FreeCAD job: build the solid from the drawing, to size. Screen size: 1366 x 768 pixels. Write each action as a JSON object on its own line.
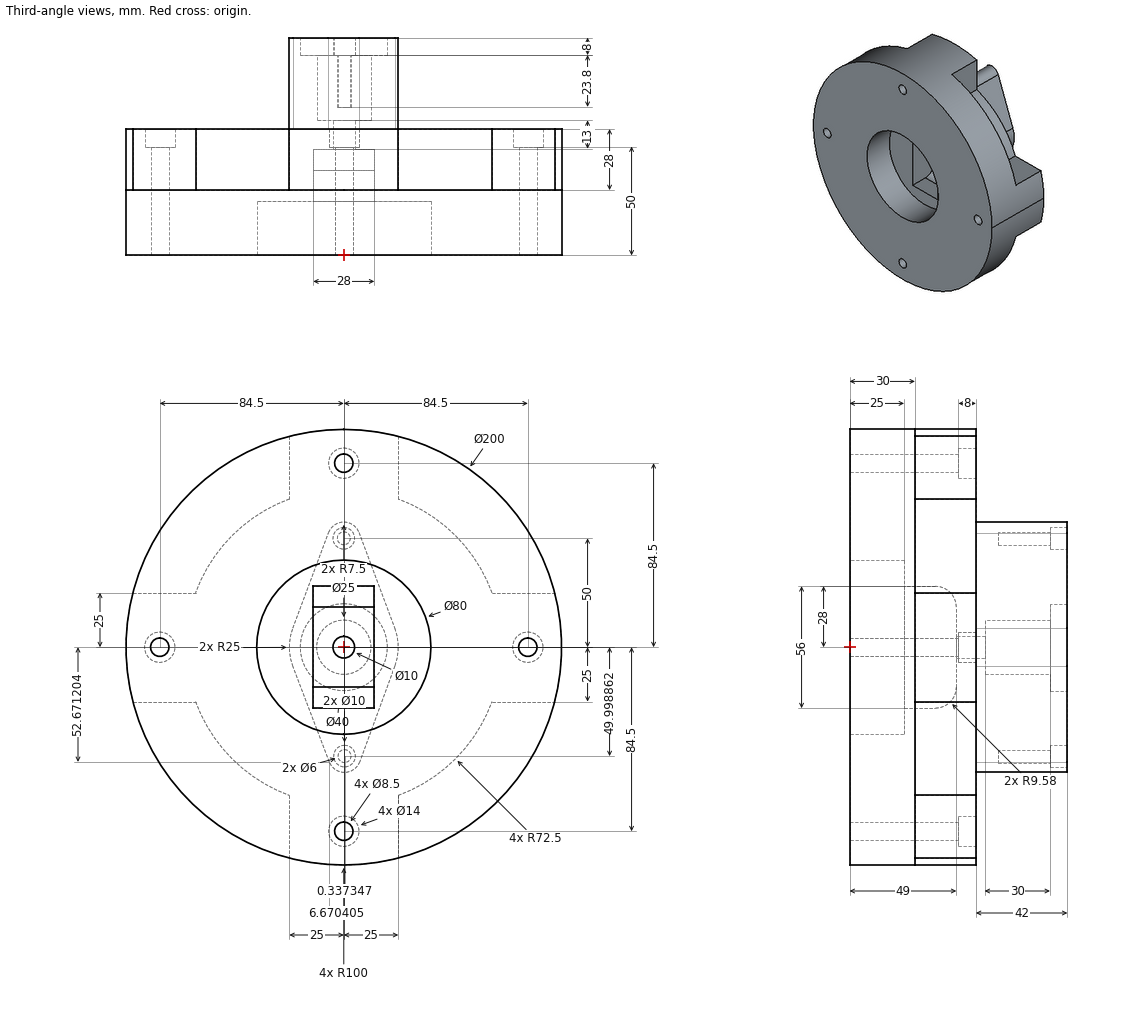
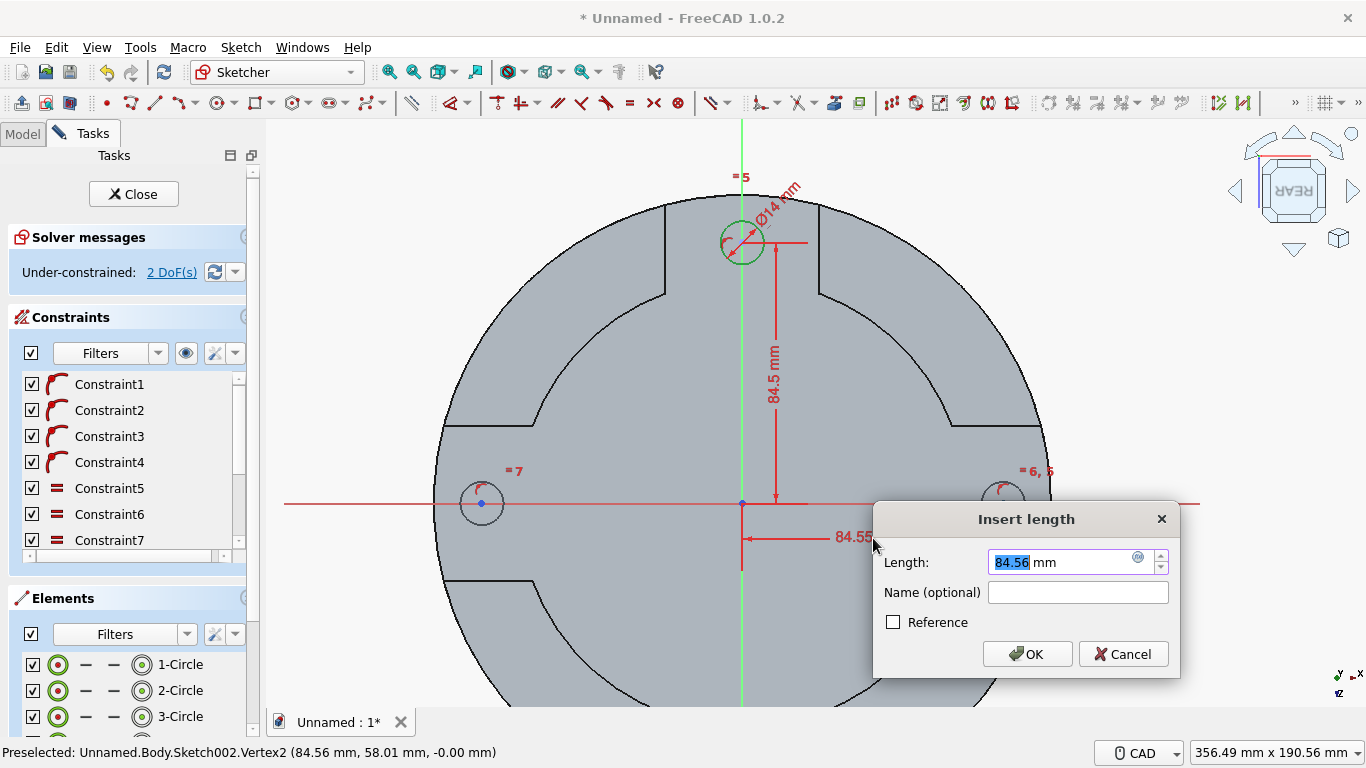
{"action": "type", "text": "84.5"}
{"action": "key", "text": "Return"}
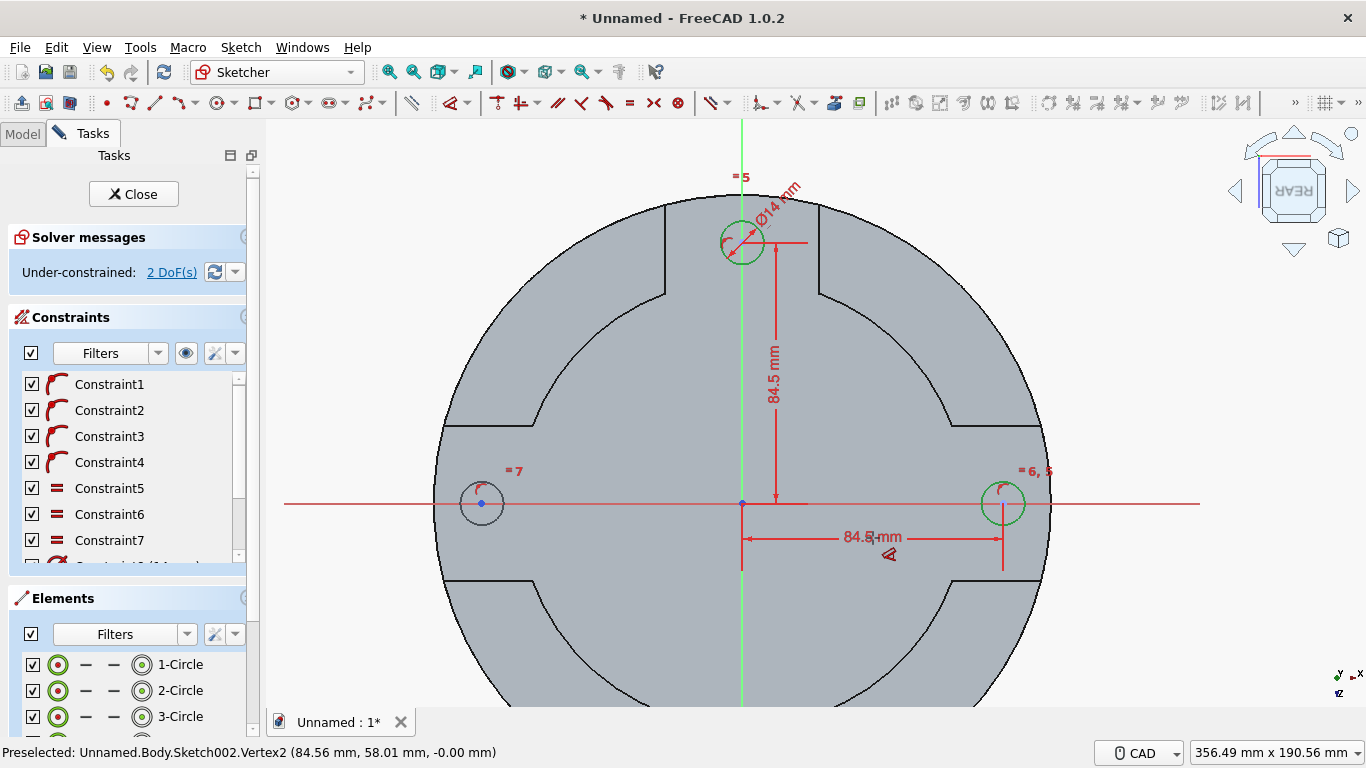
{"action": "scroll", "coordinate": [758, 229], "scroll_direction": "down", "scroll_amount": 2}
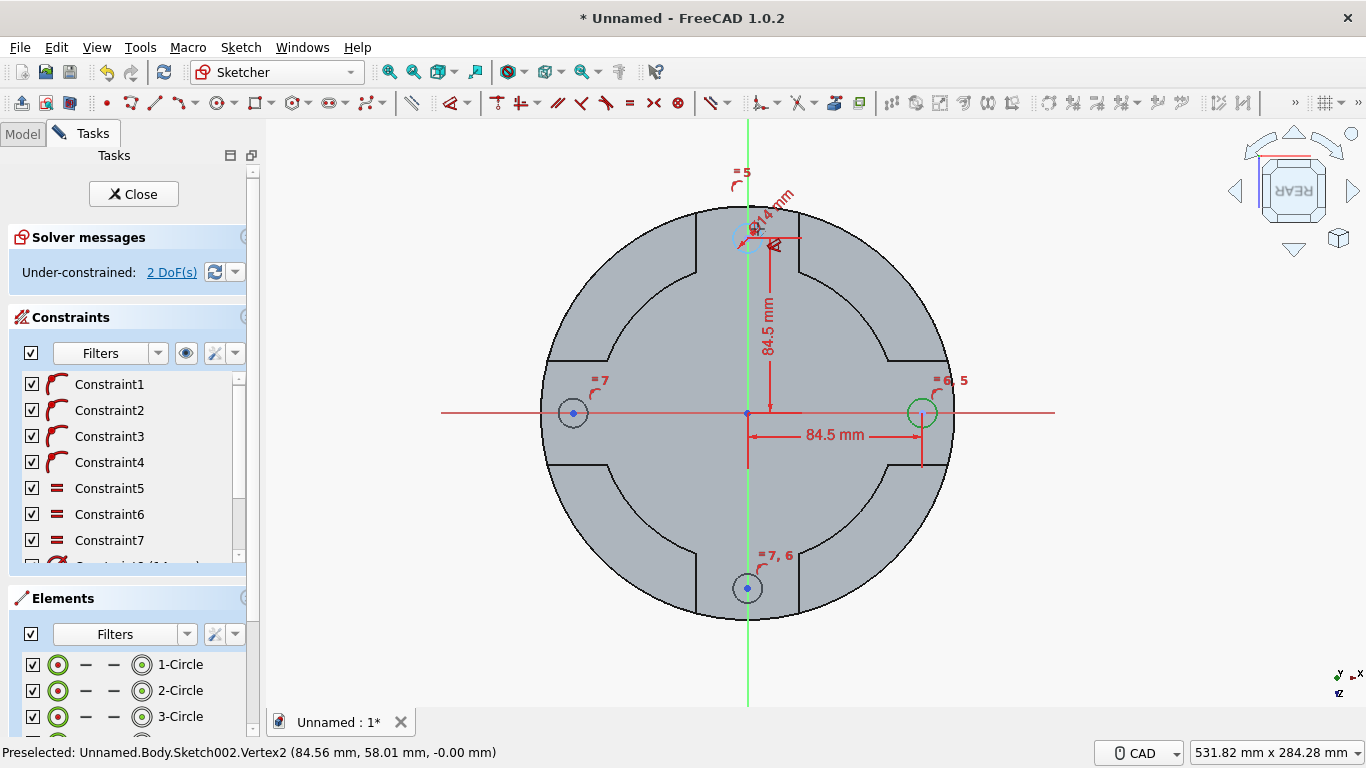
{"action": "left_click", "coordinate": [748, 588]}
{"action": "left_click", "coordinate": [782, 501]}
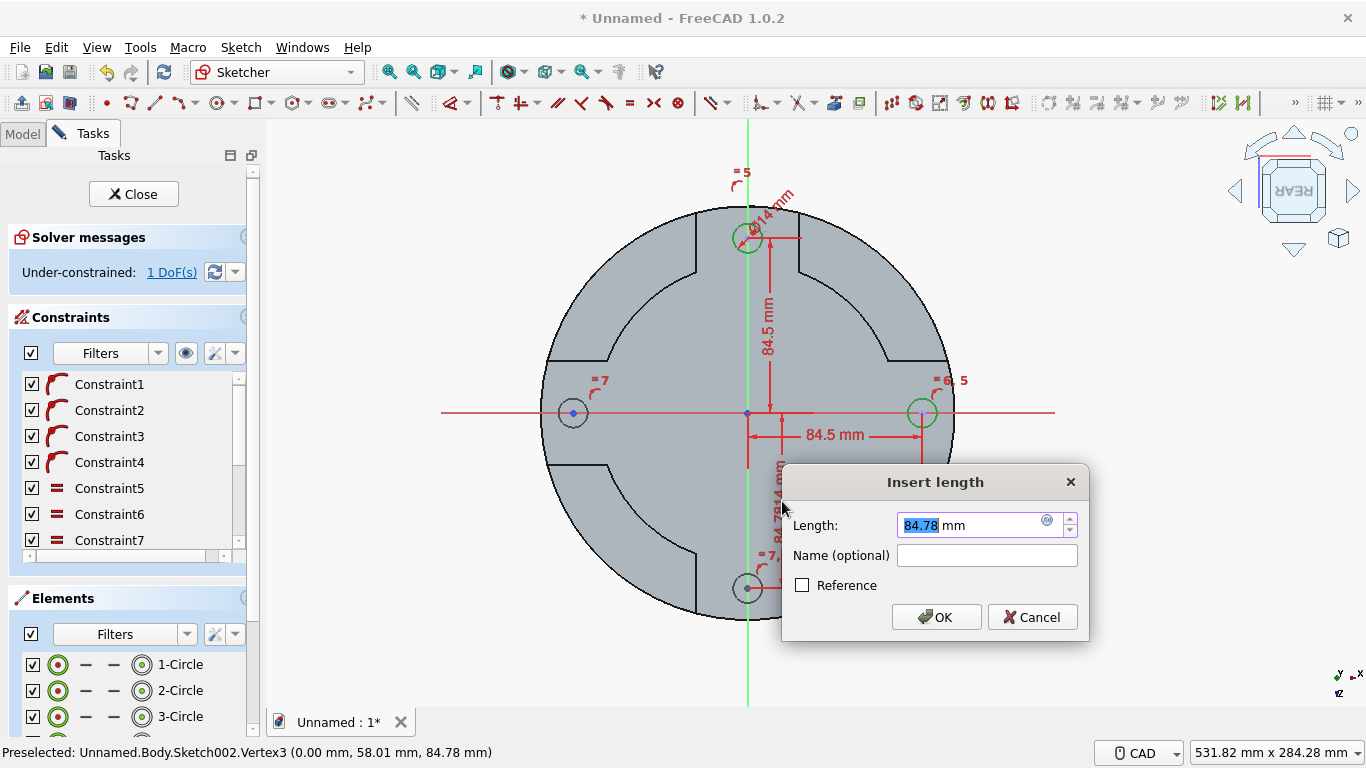
{"action": "type", "text": "84.5"}
{"action": "key", "text": "Return"}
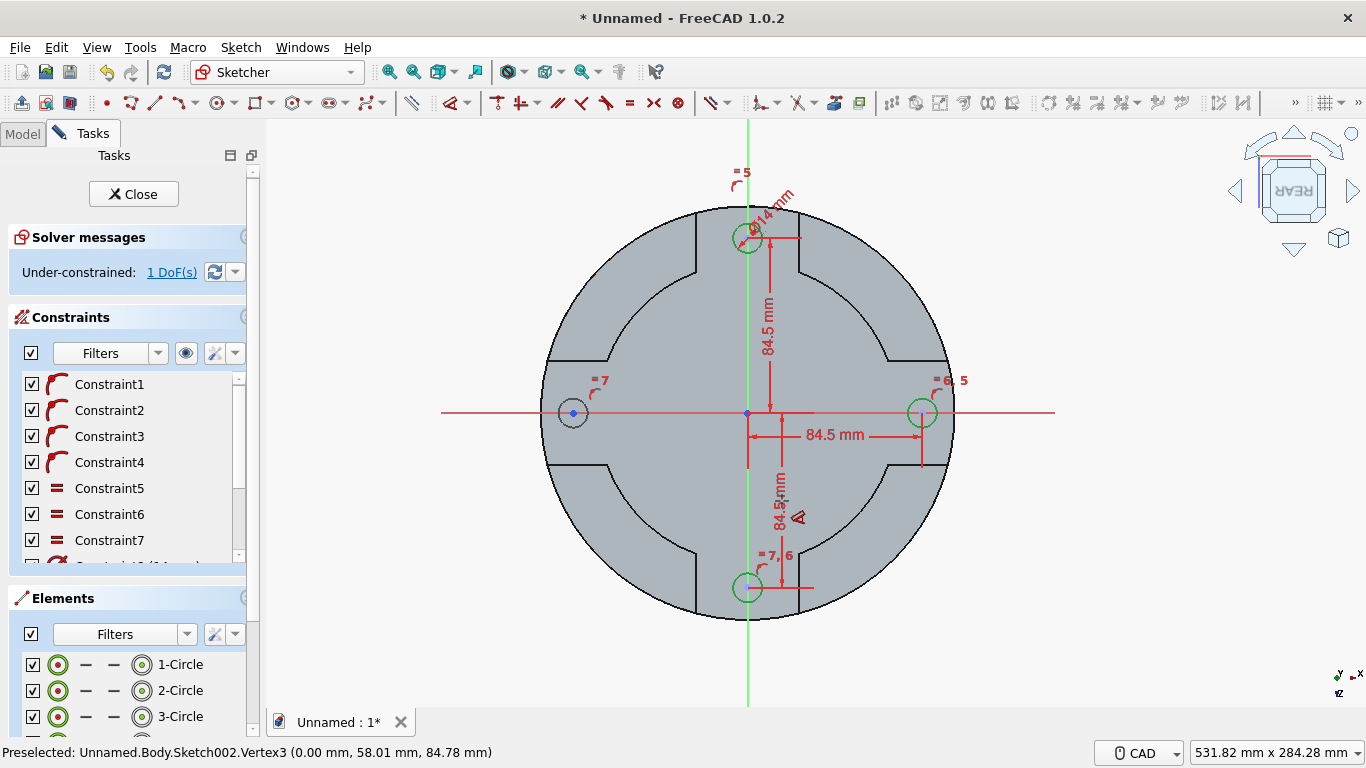
{"action": "left_click", "coordinate": [573, 413]}
{"action": "left_click", "coordinate": [660, 447]}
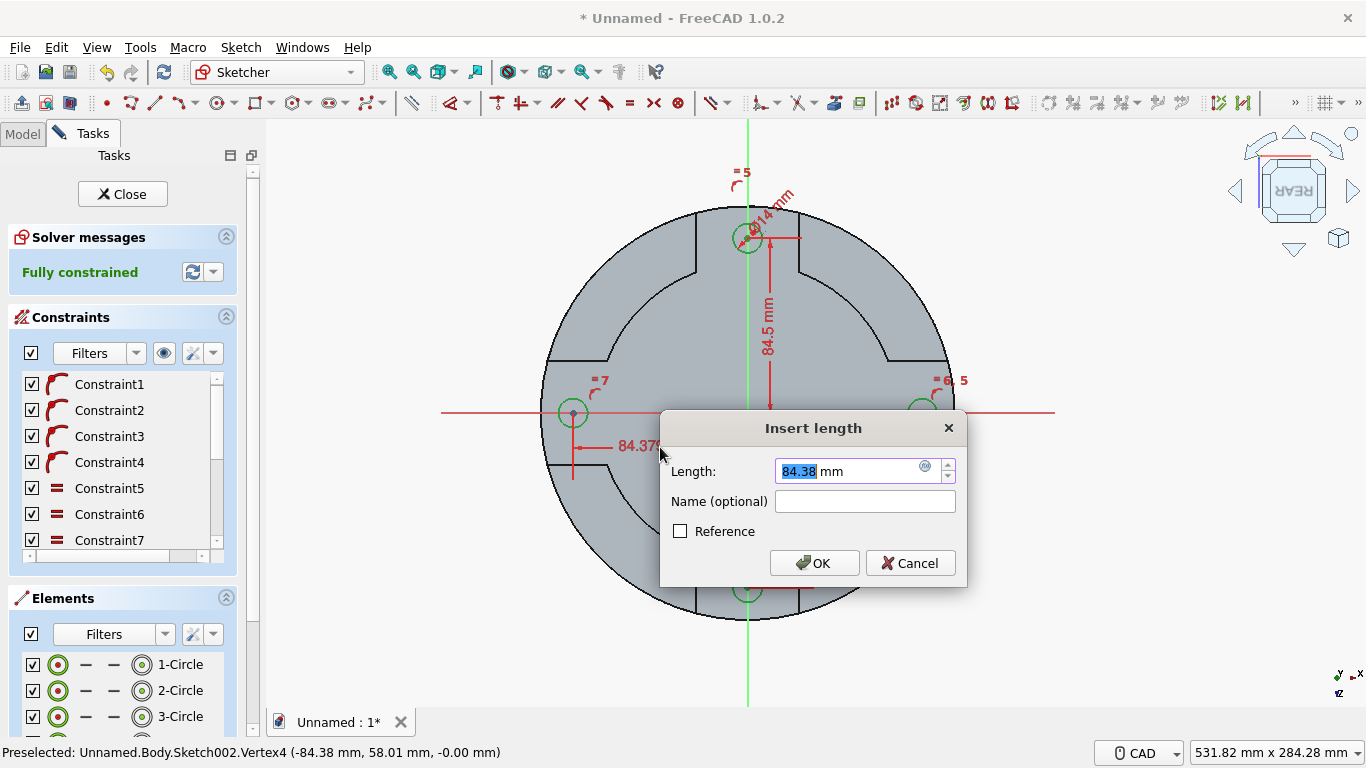
{"action": "type", "text": "84.5"}
{"action": "key", "text": "Return"}
{"action": "key", "text": "Escape"}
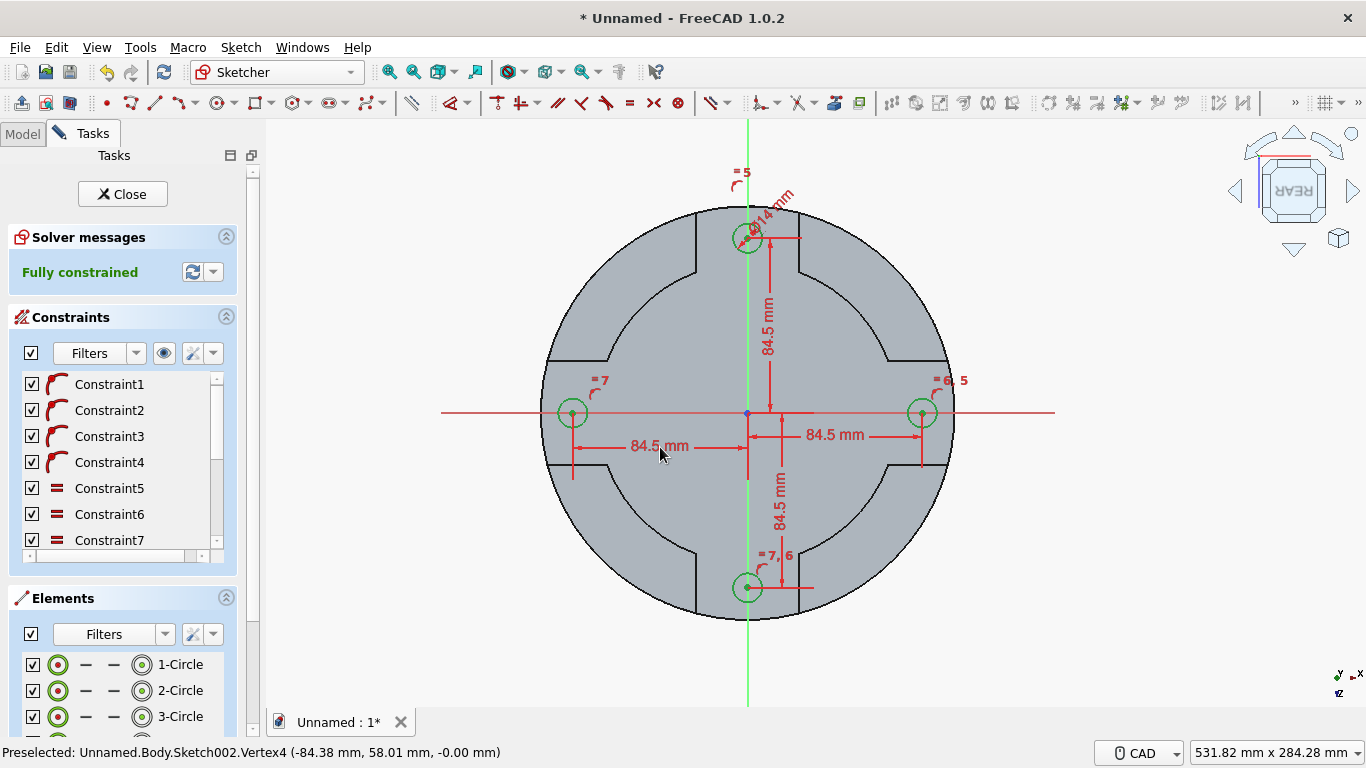
{"action": "left_click", "coordinate": [123, 194]}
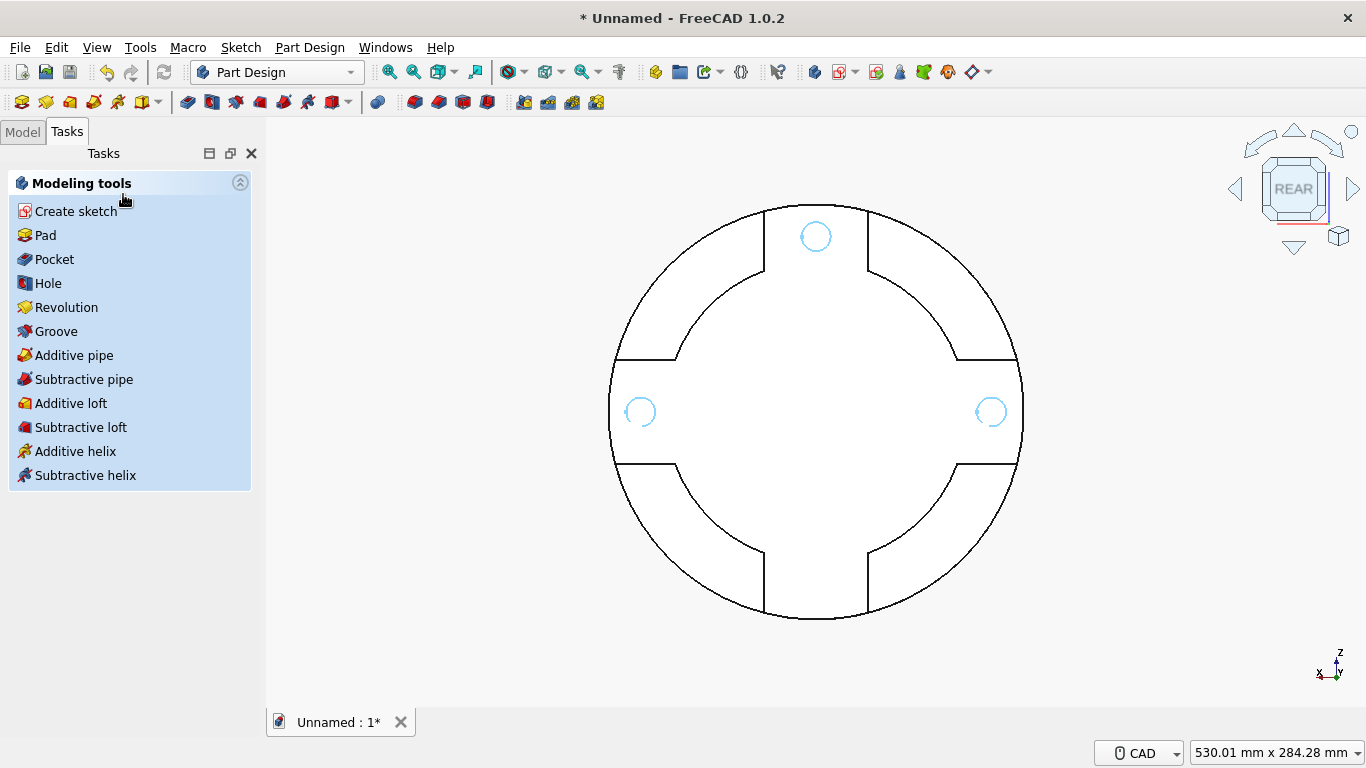
{"action": "left_click", "coordinate": [188, 102]}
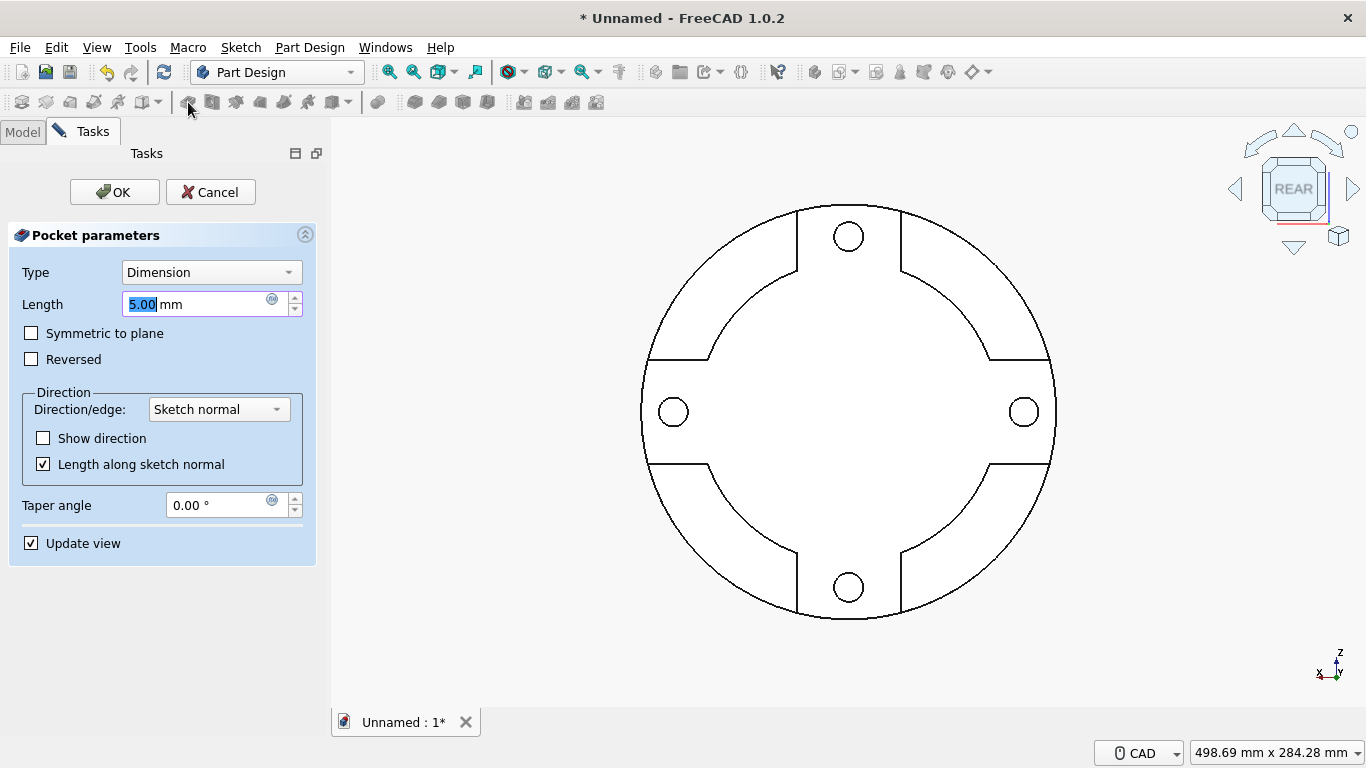
{"action": "type", "text": "8"}
{"action": "key", "text": "Tab"}